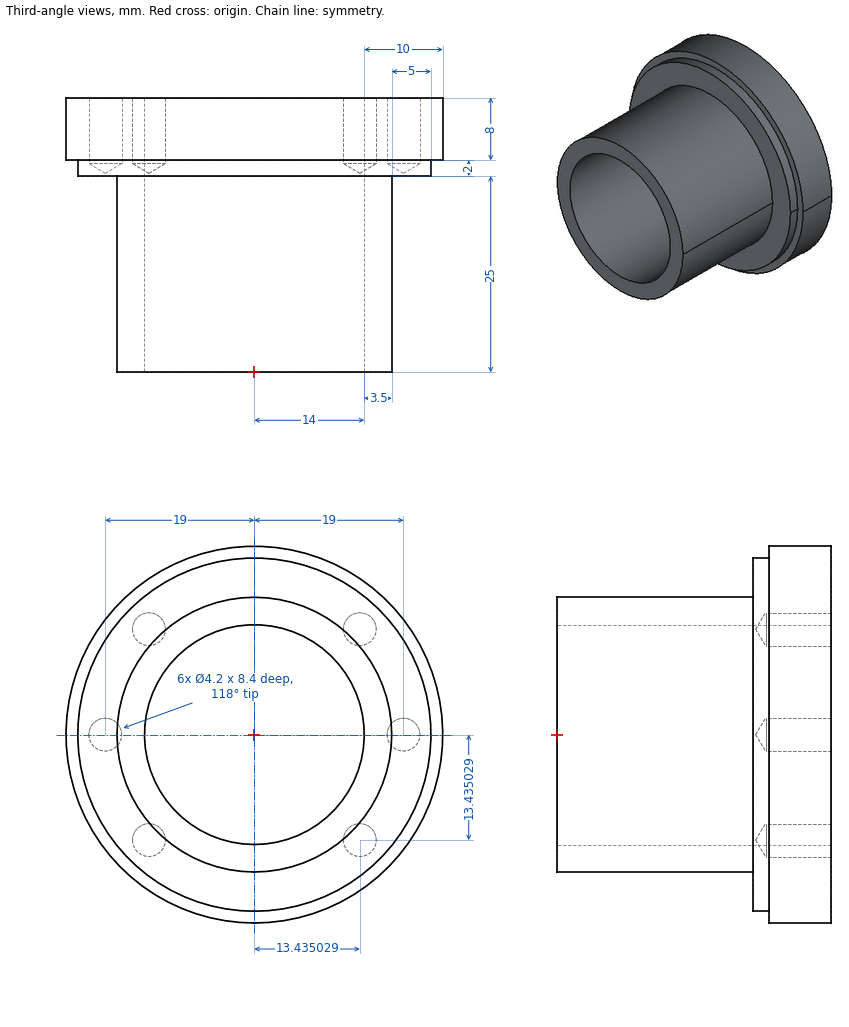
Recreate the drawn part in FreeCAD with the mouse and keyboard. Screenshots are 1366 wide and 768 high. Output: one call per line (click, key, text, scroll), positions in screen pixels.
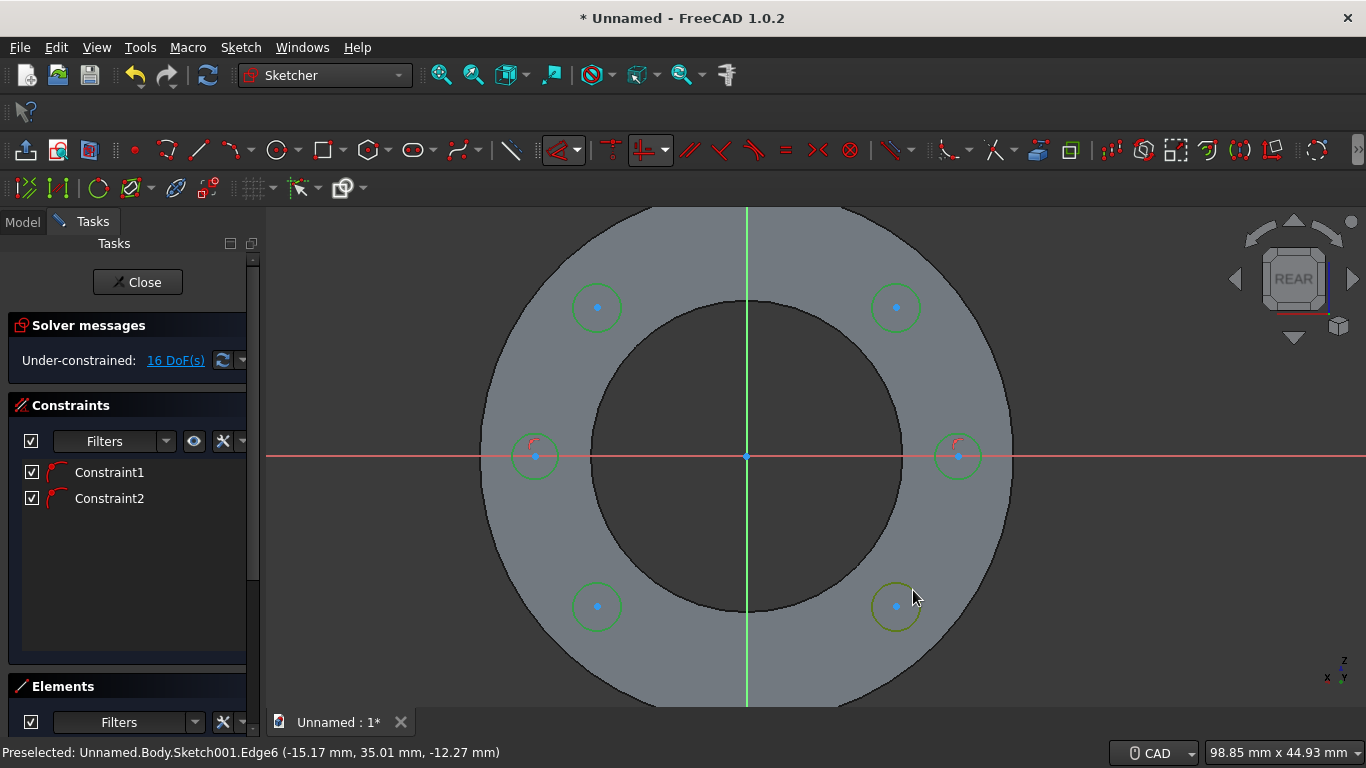
click(786, 150)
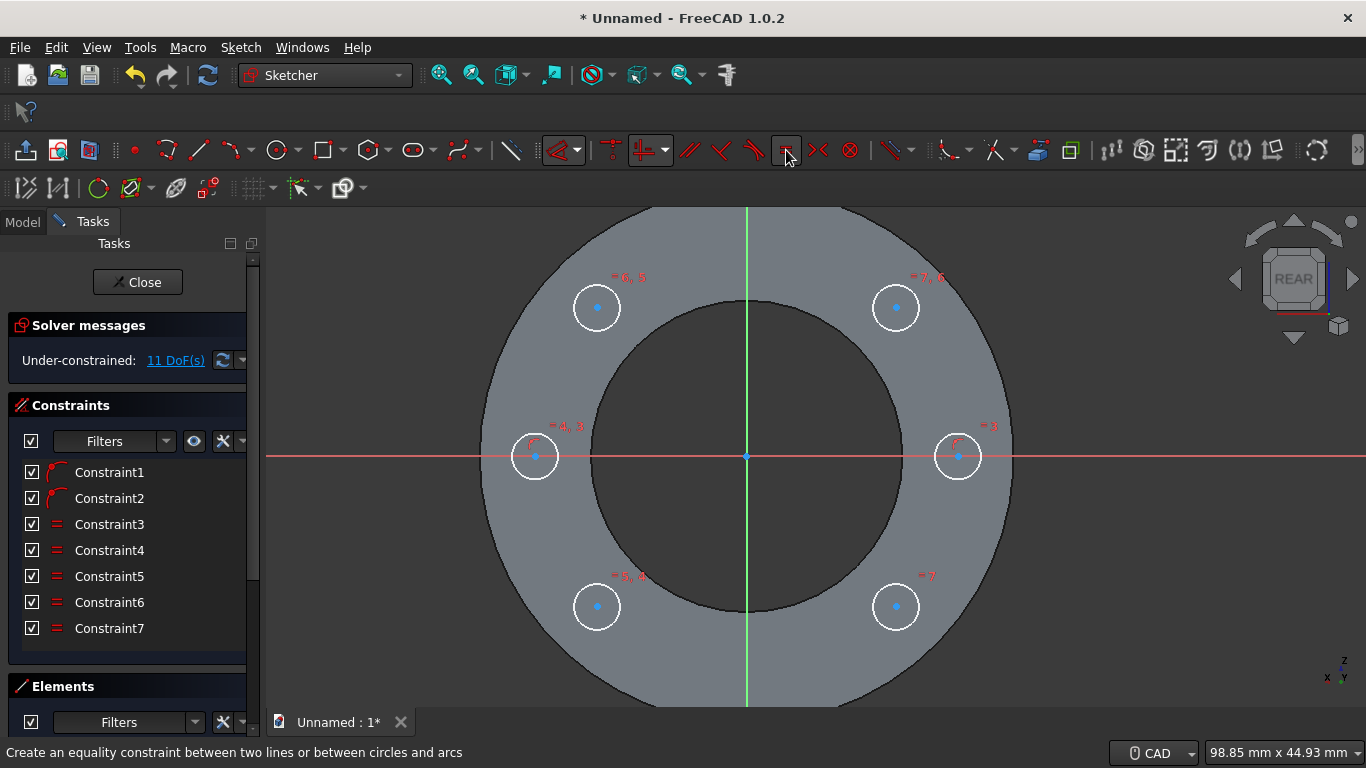
click(597, 607)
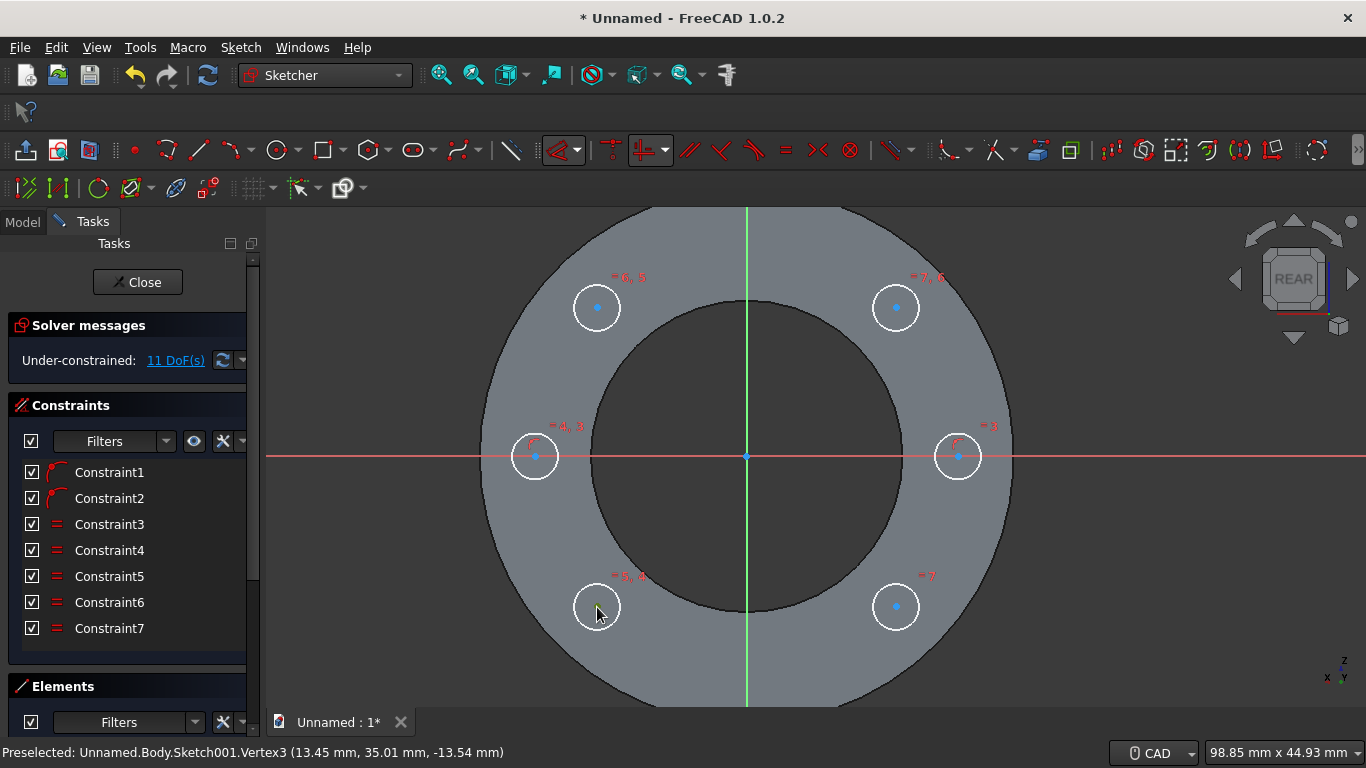
click(597, 308)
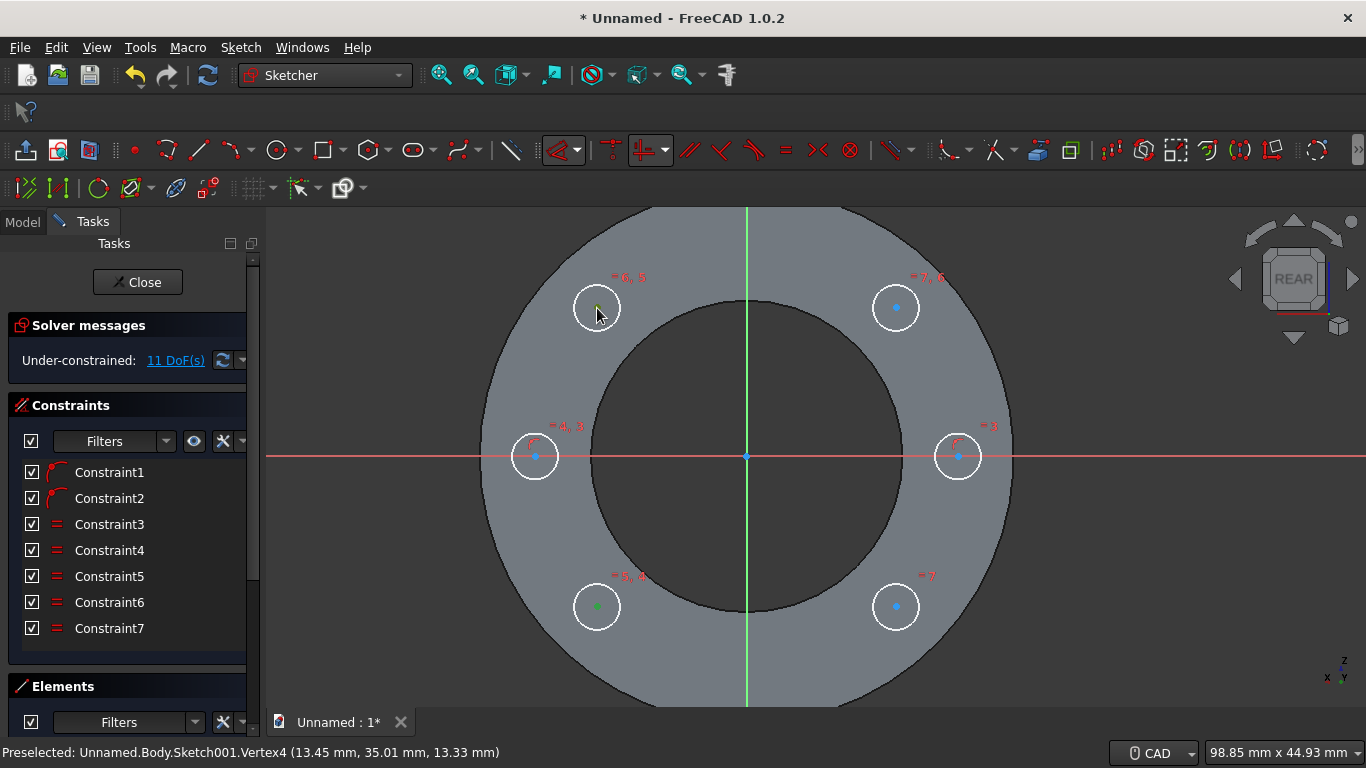
click(359, 456)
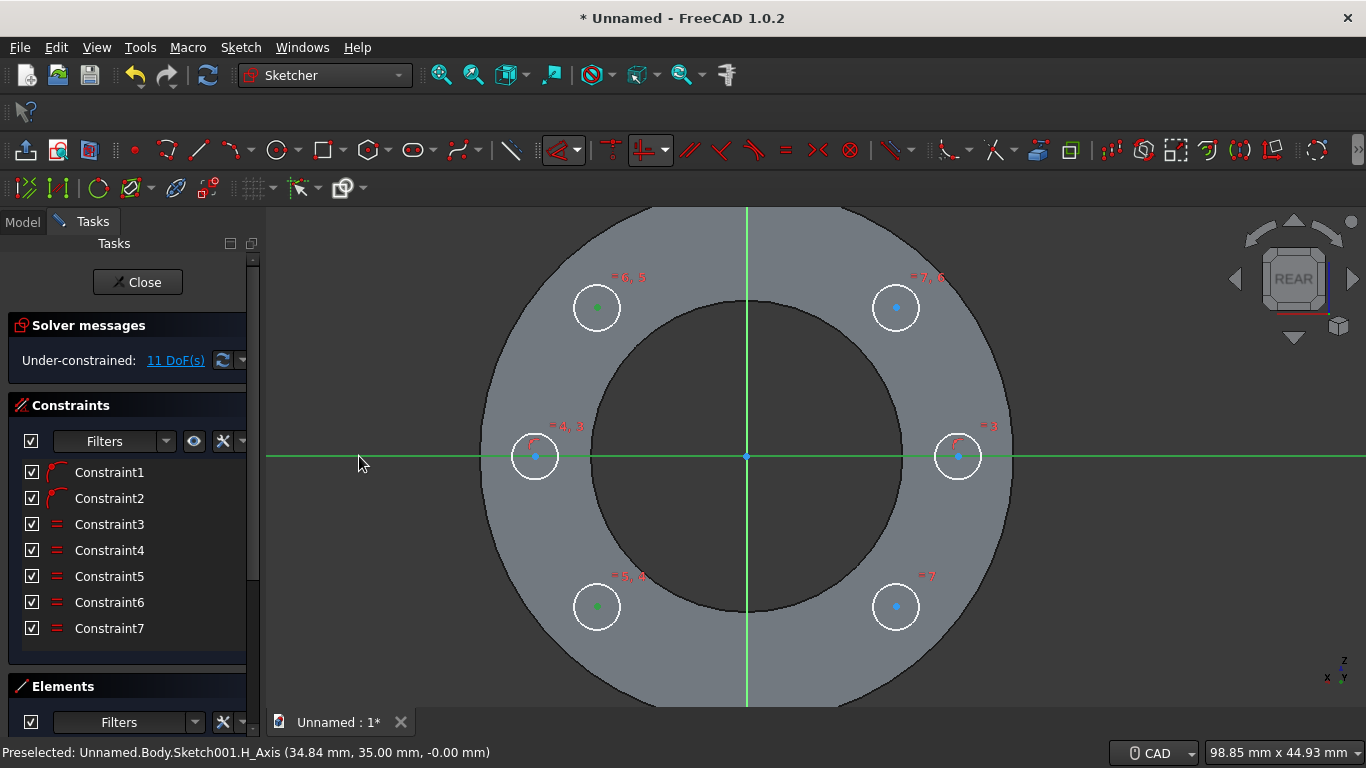
click(818, 150)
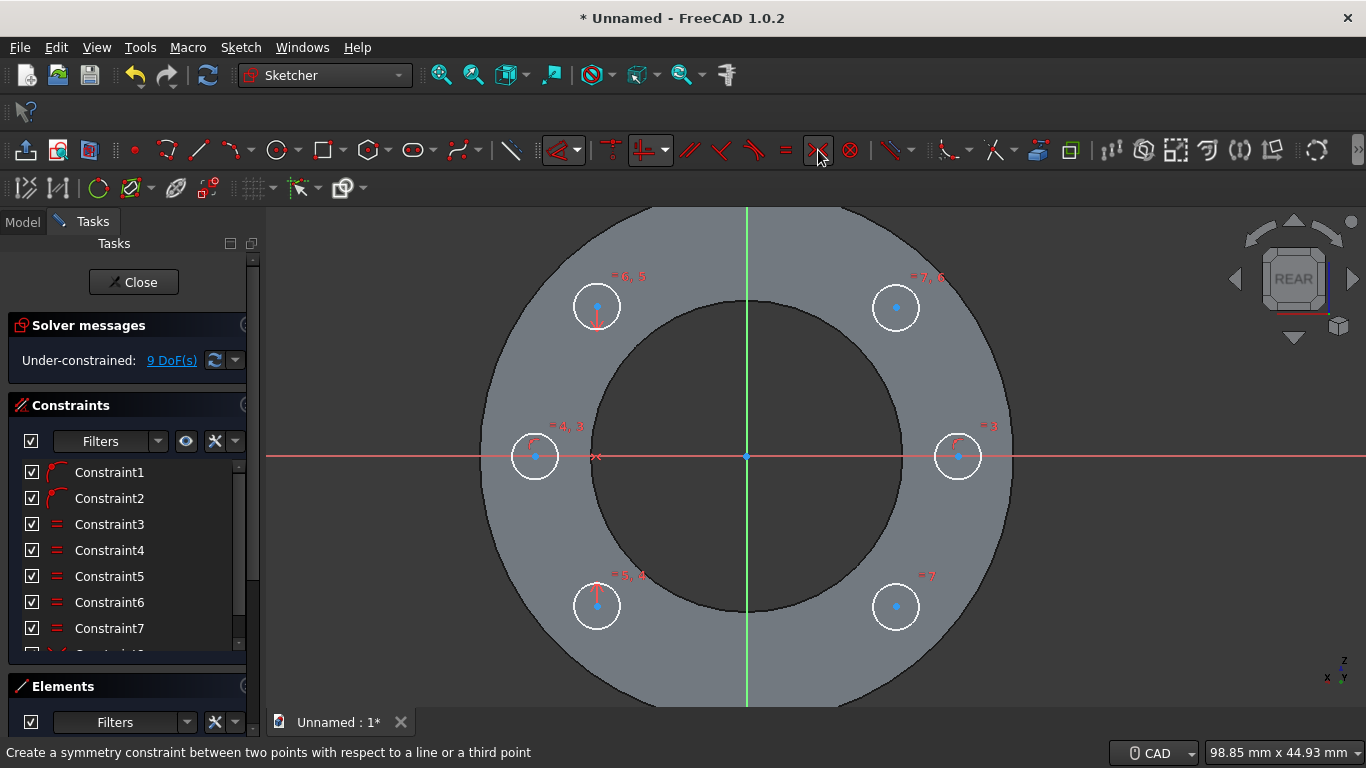
click(597, 307)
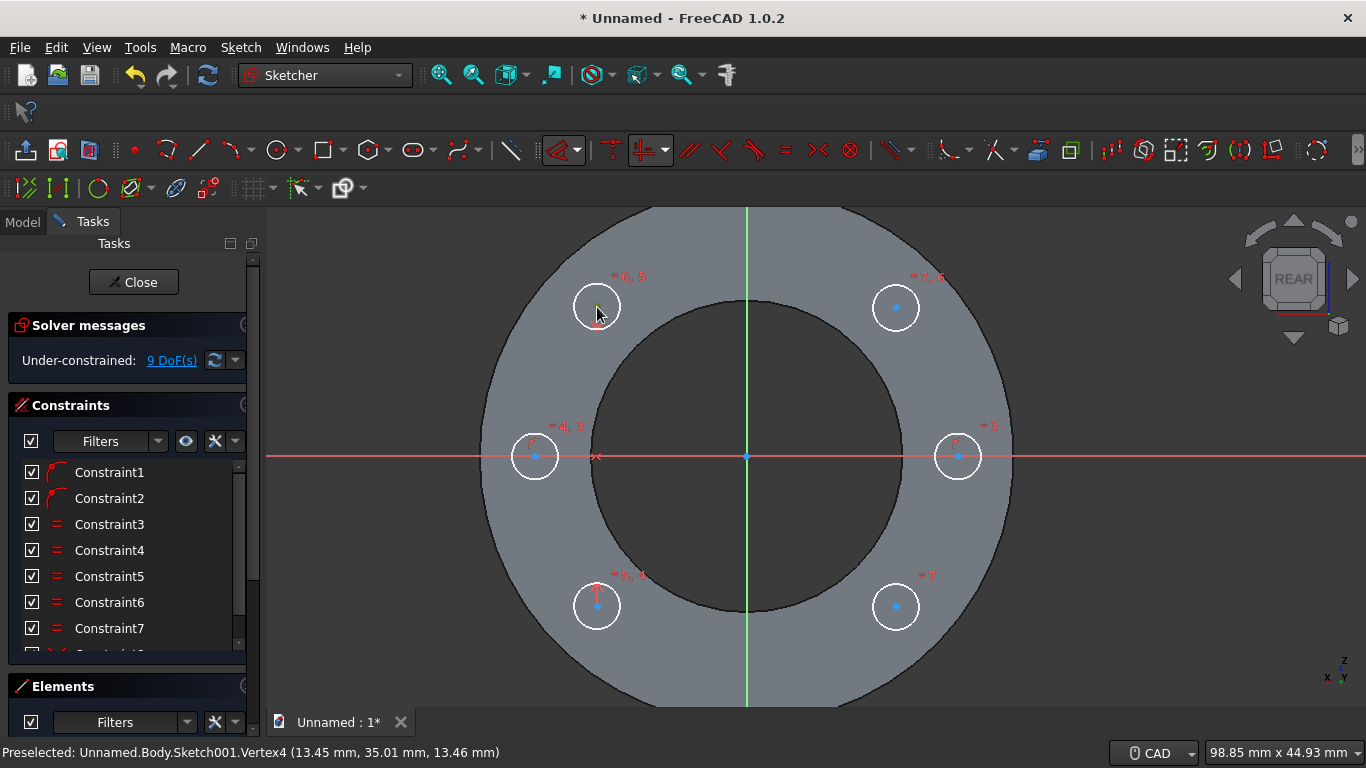
click(896, 308)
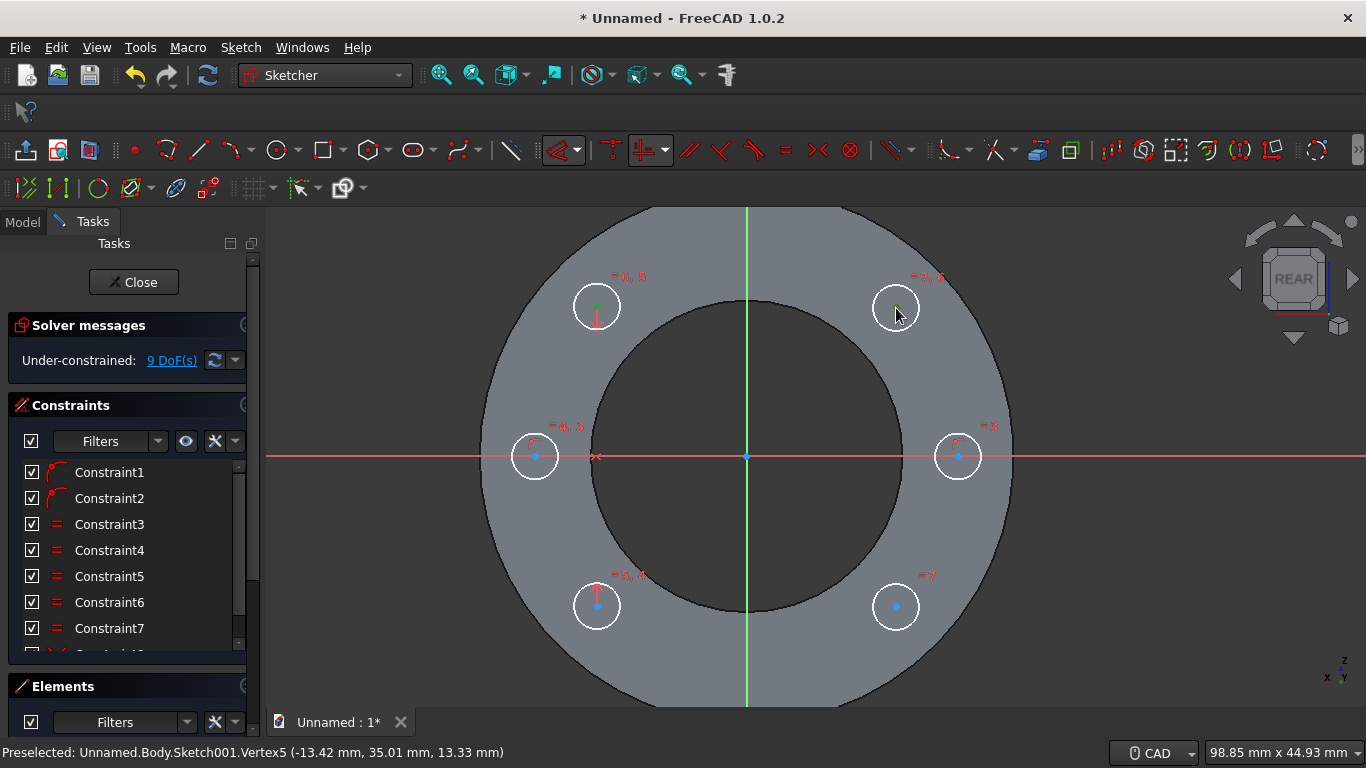
click(747, 647)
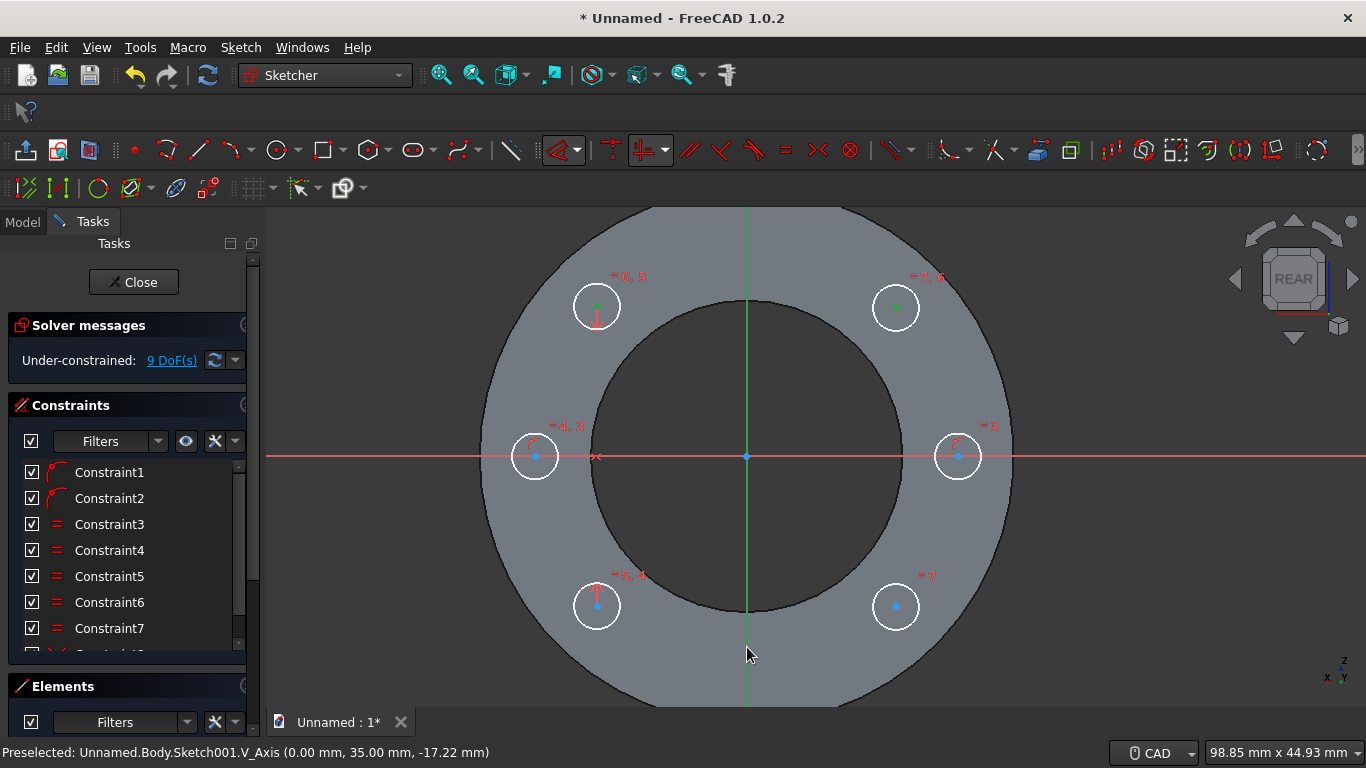
click(818, 150)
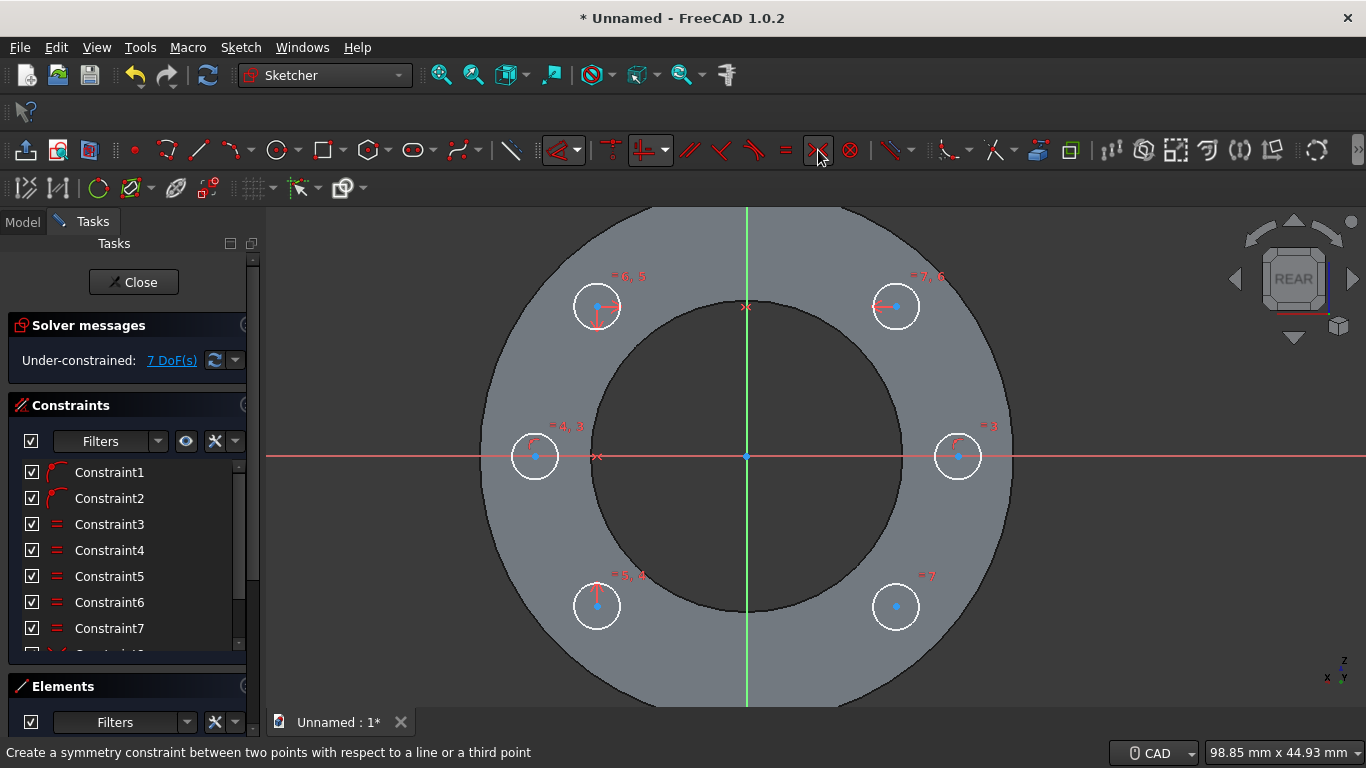
click(597, 606)